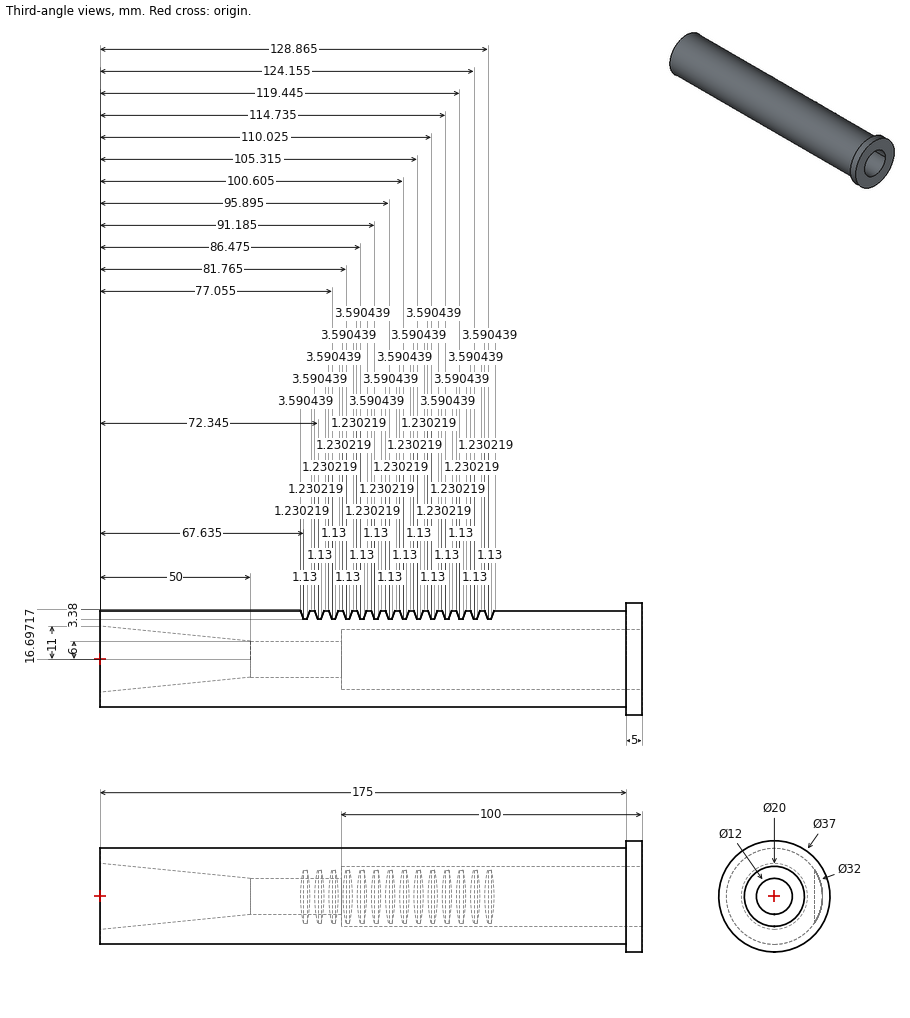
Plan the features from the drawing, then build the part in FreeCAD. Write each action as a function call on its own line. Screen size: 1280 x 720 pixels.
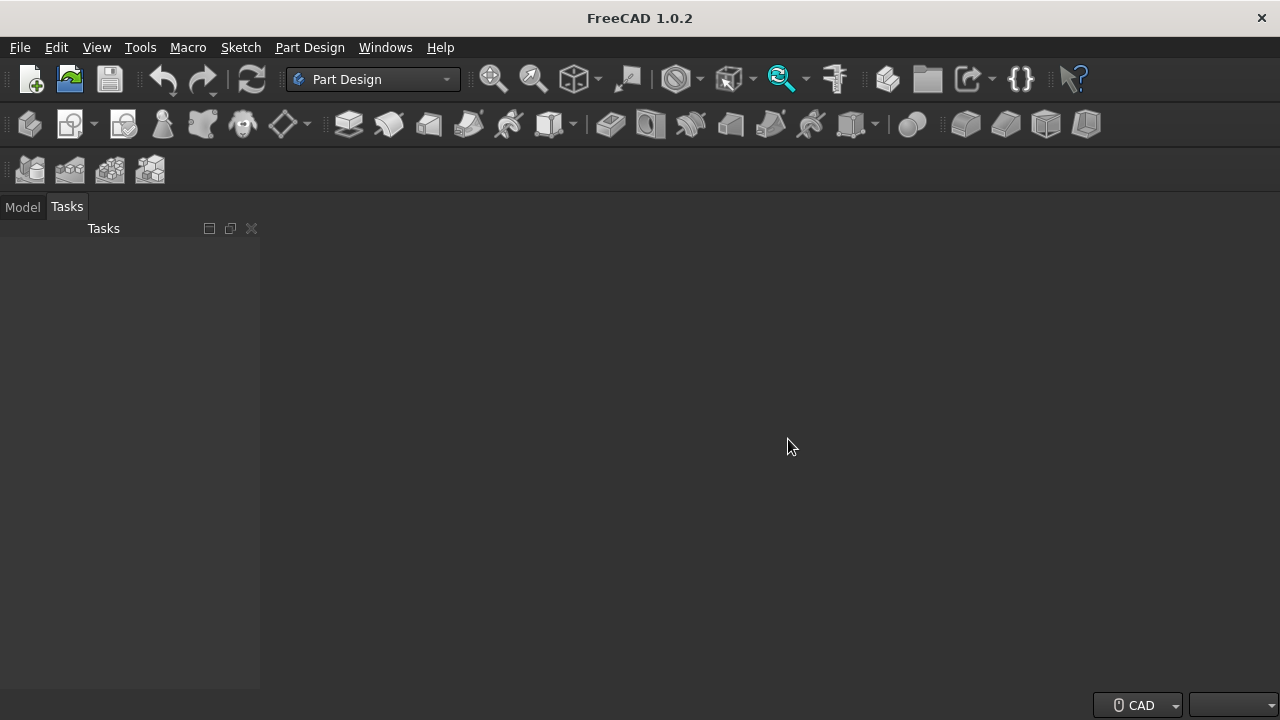
key(ctrl+n)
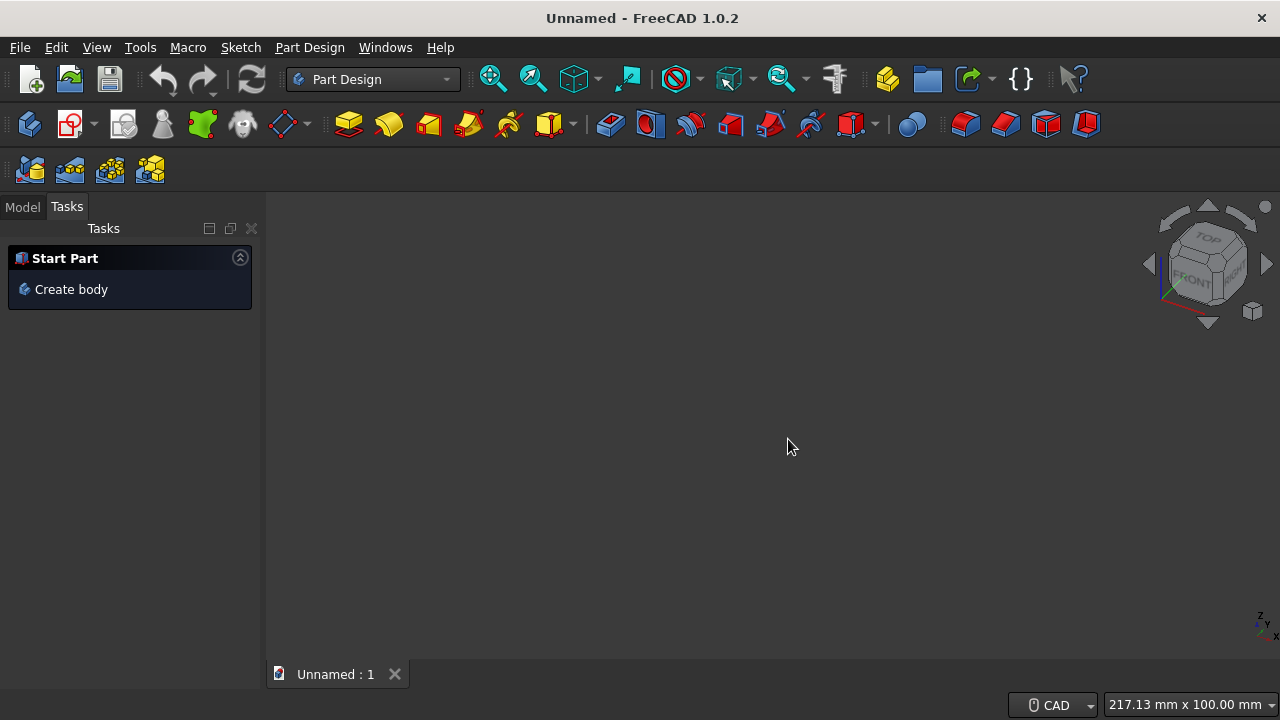
click(70, 124)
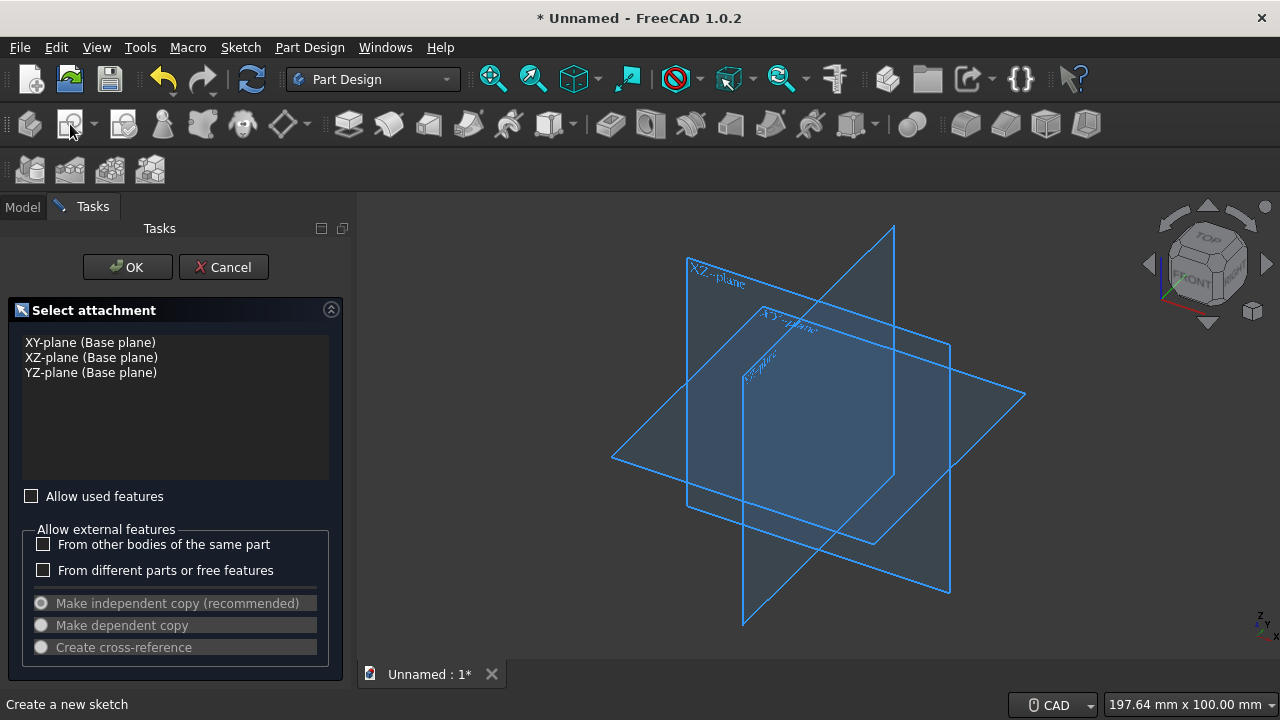
click(82, 372)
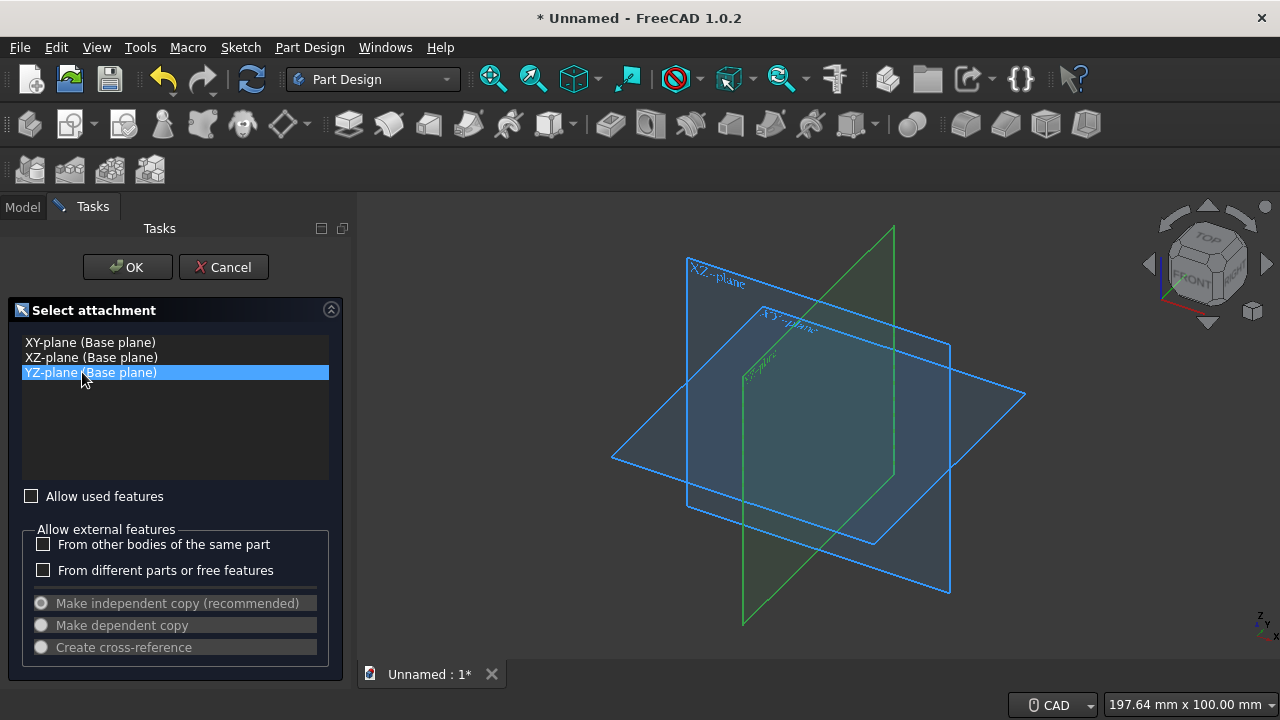
click(128, 267)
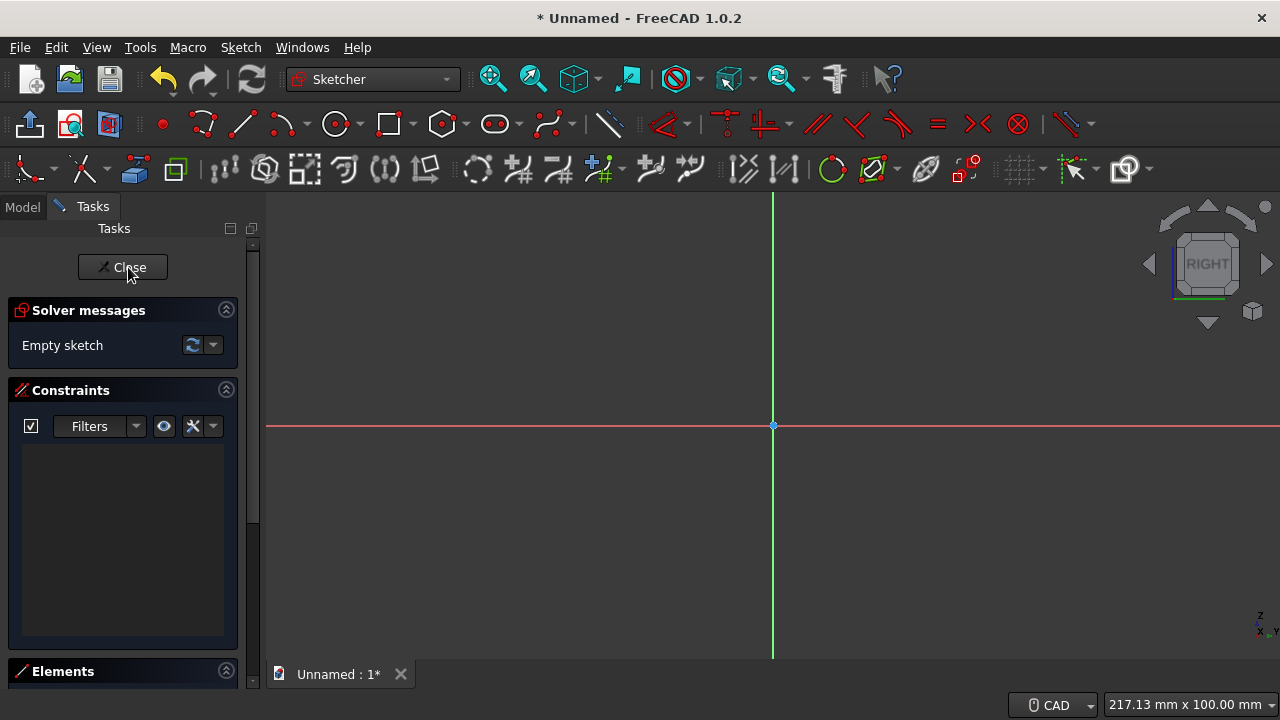
scroll(856, 426, up, 3)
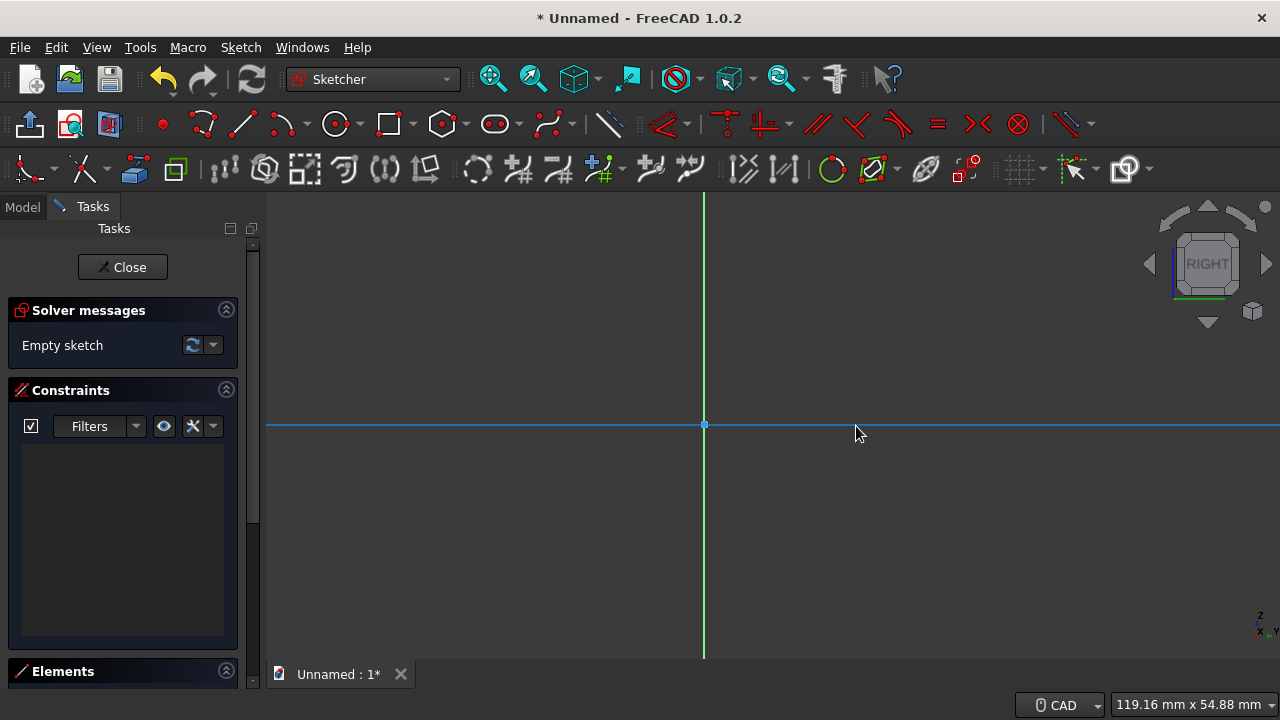
key(g)
key(c)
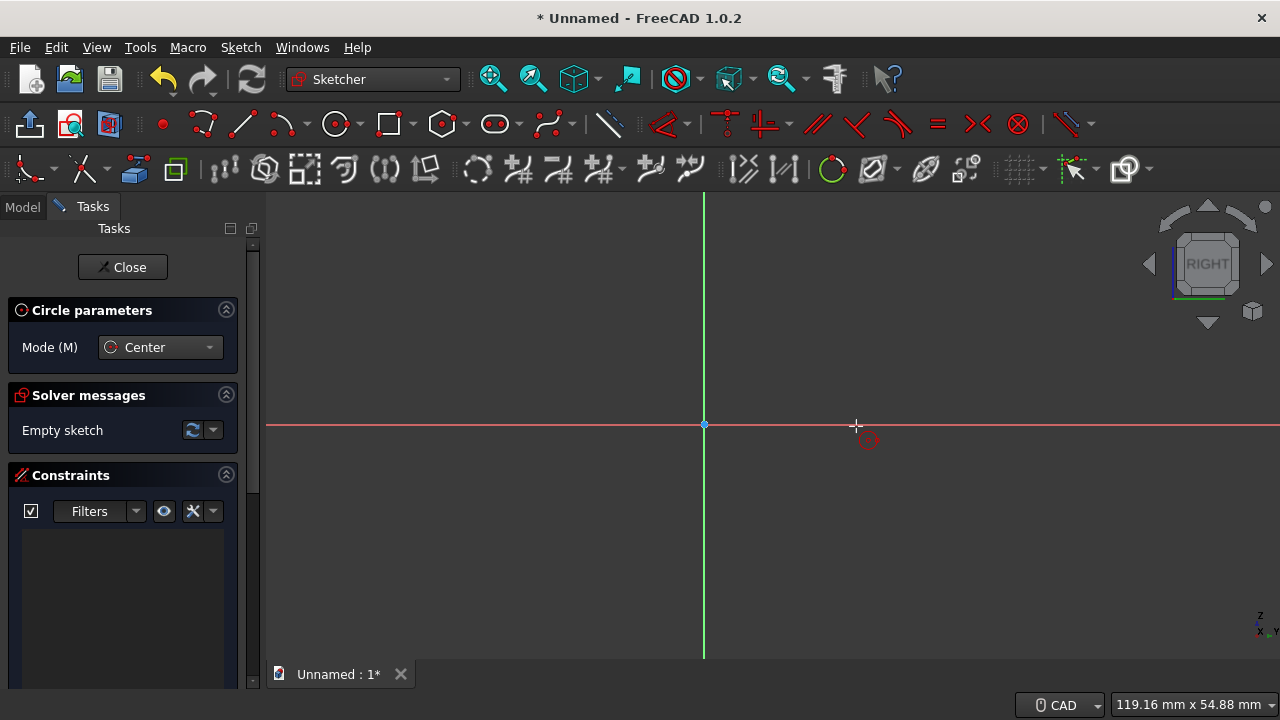
click(704, 425)
move(801, 328)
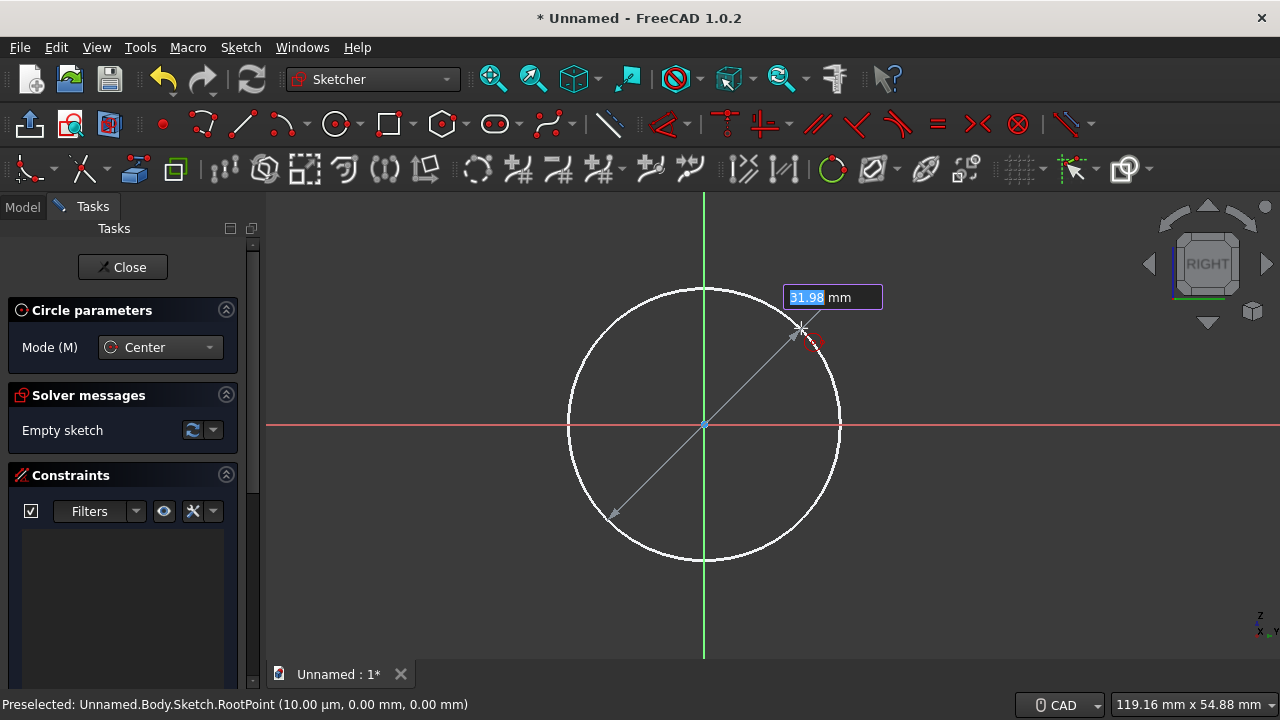
text(32)
key(Return)
key(Escape)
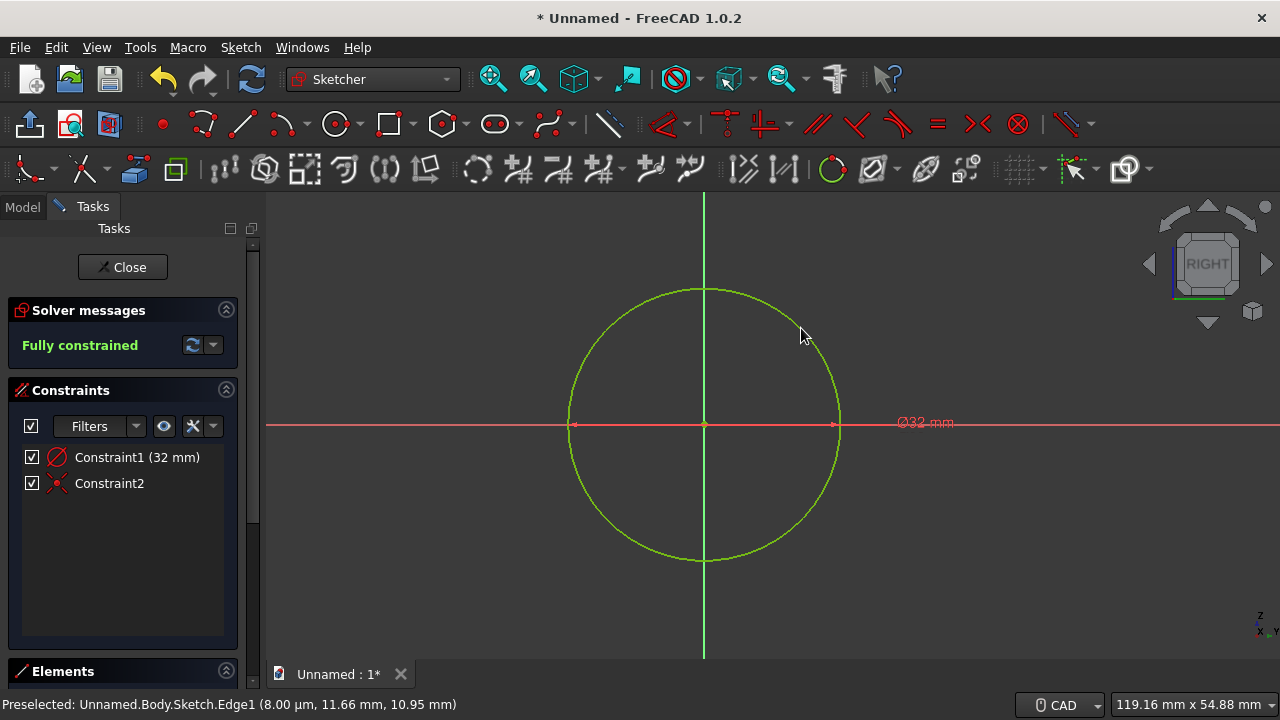
click(123, 267)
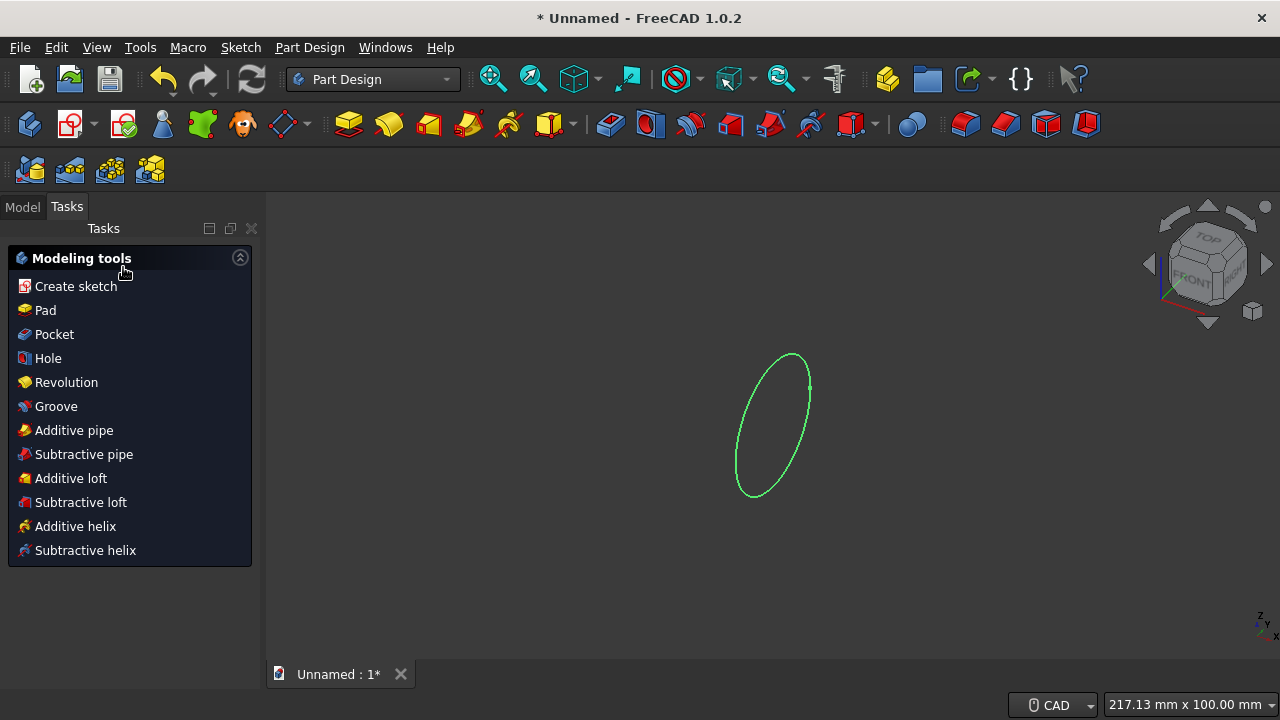
click(350, 124)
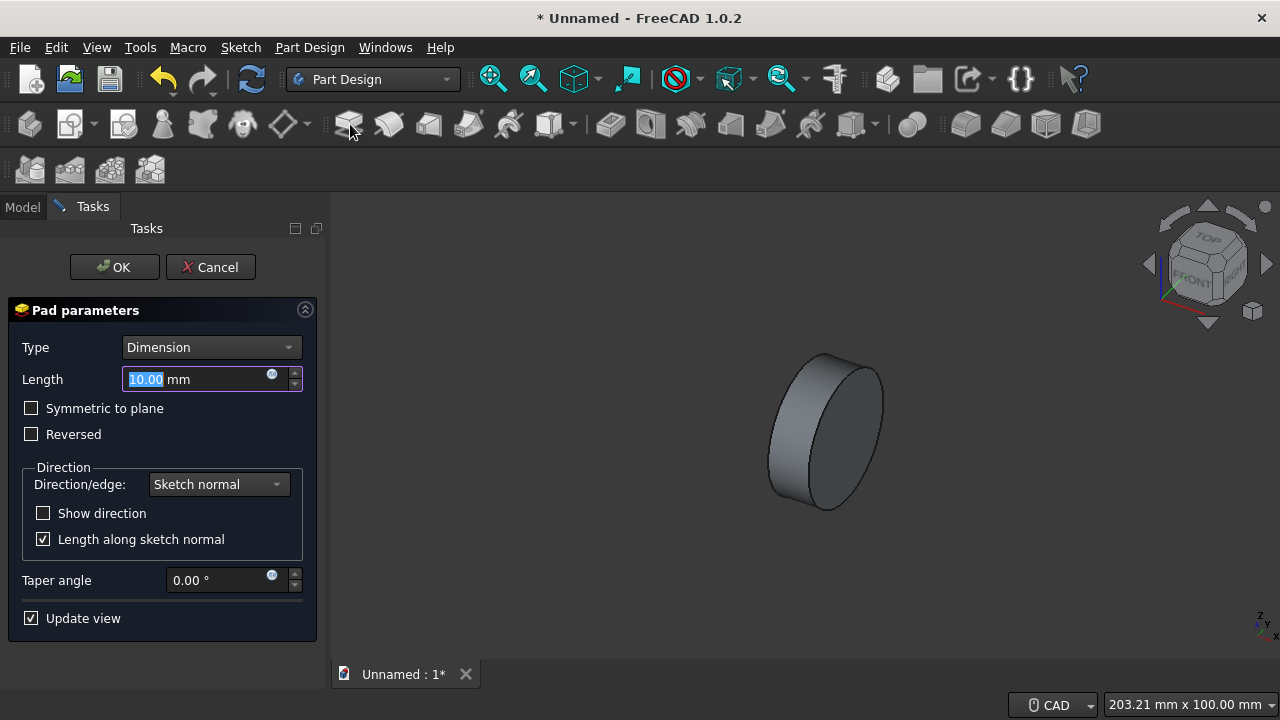
text(175)
key(Tab)